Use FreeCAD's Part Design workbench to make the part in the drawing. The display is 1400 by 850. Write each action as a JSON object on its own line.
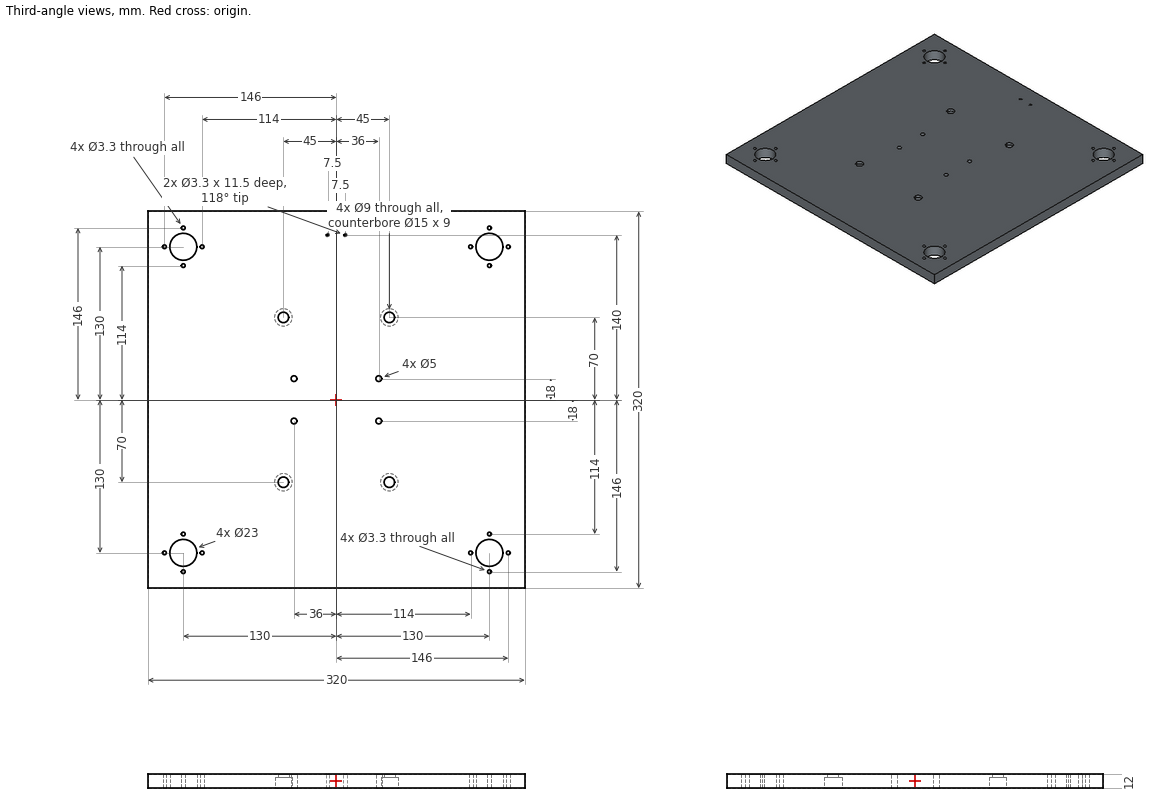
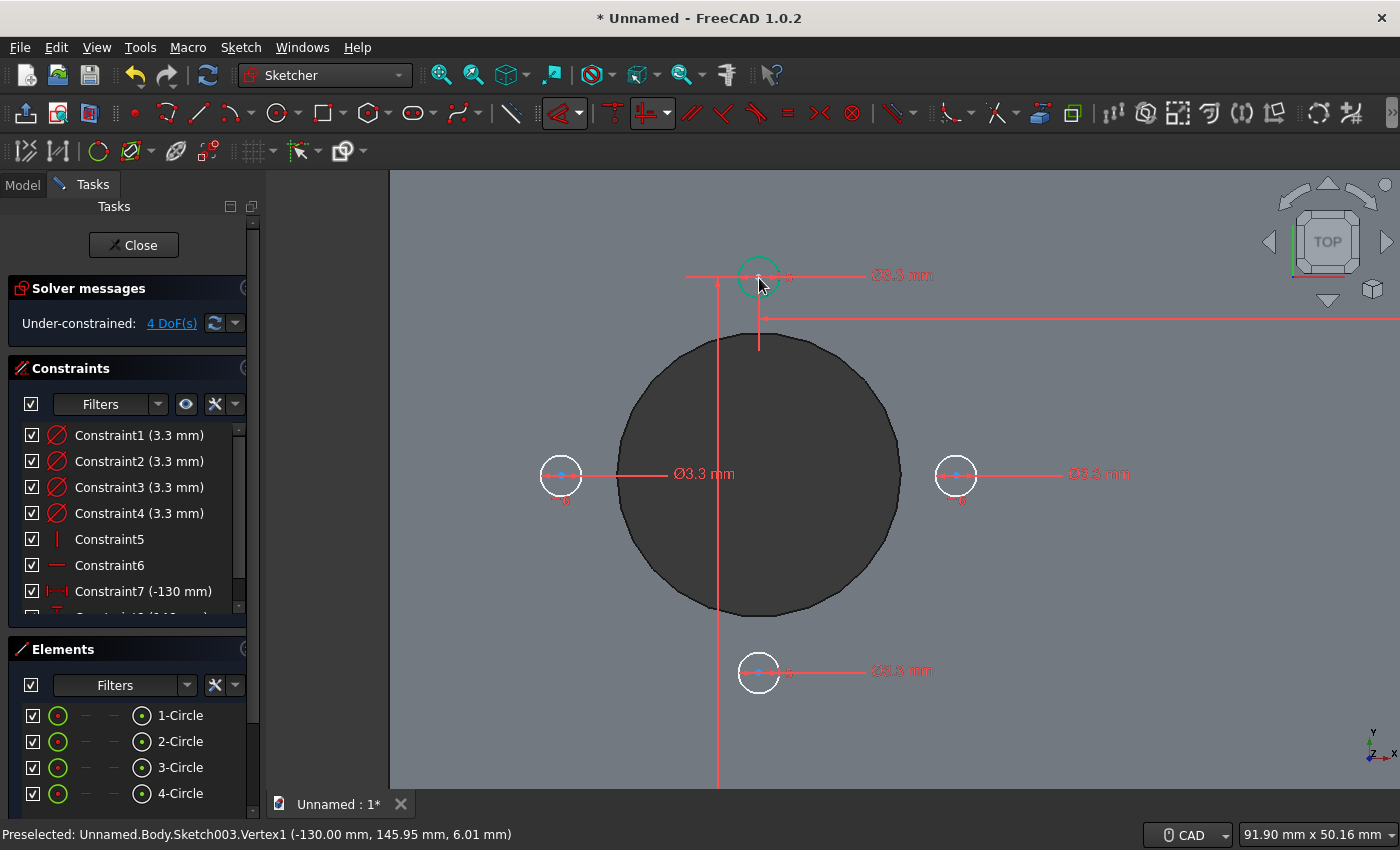
{"action": "left_click", "coordinate": [956, 476]}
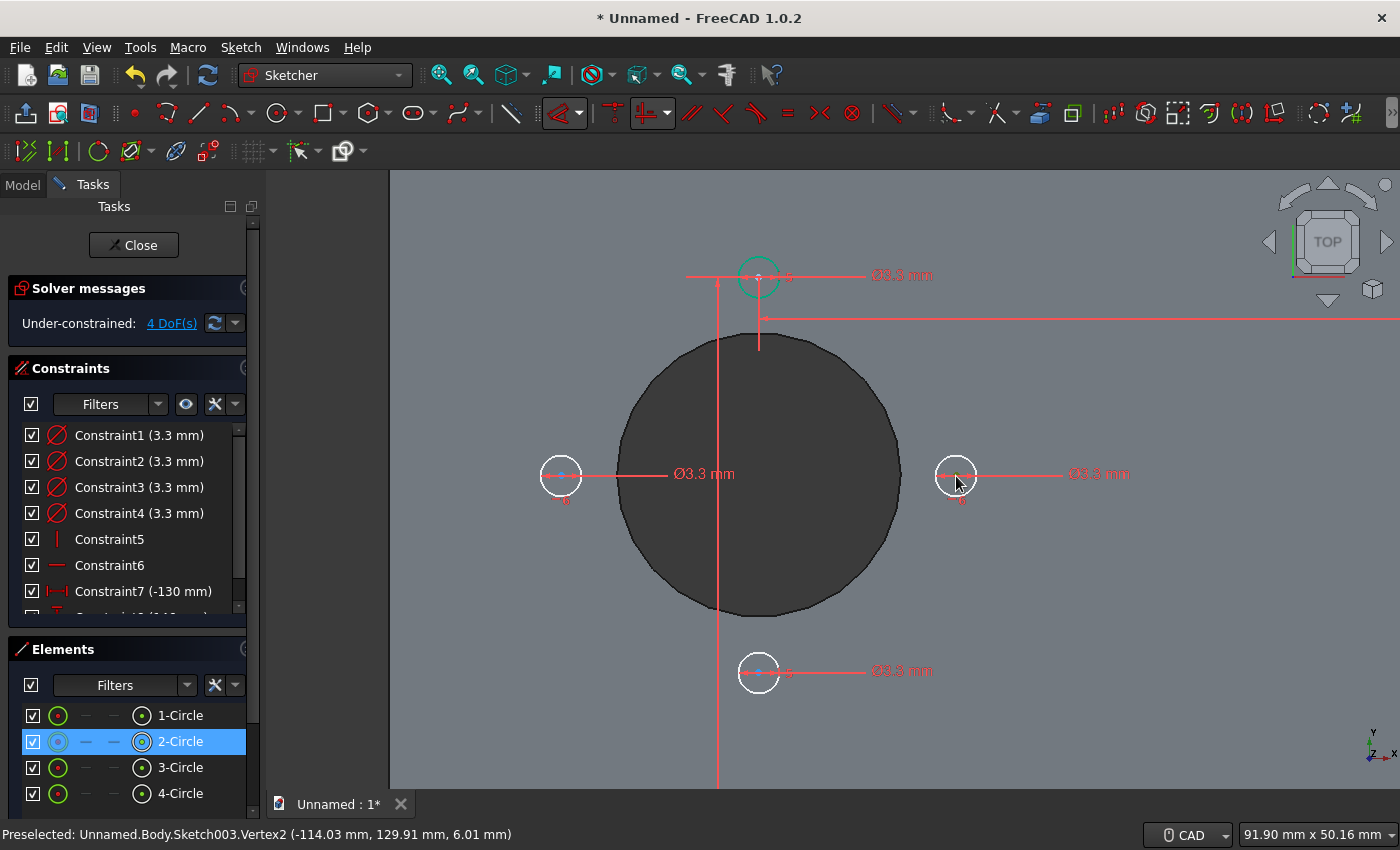
{"action": "left_click", "coordinate": [582, 114]}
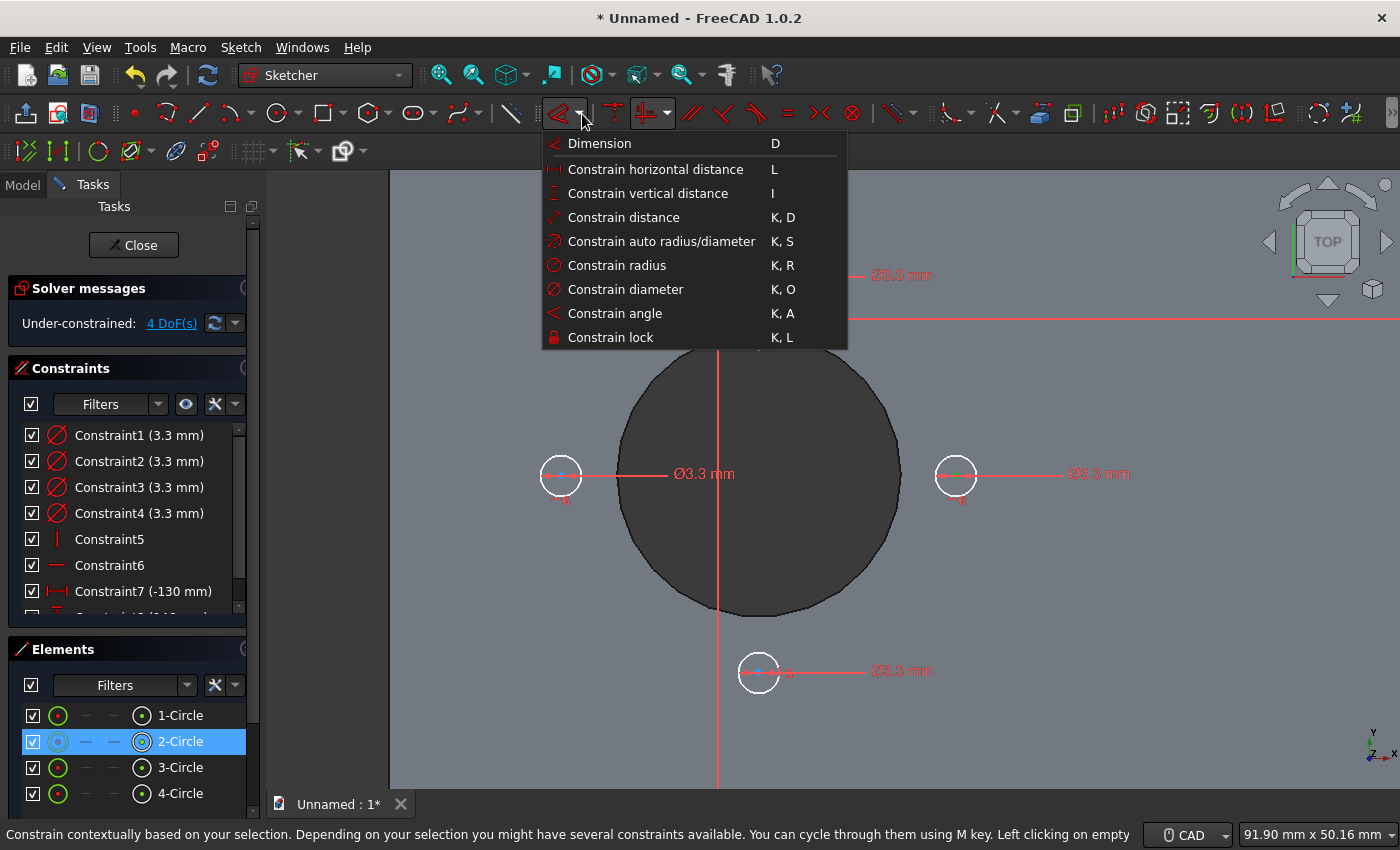
{"action": "left_click", "coordinate": [695, 169]}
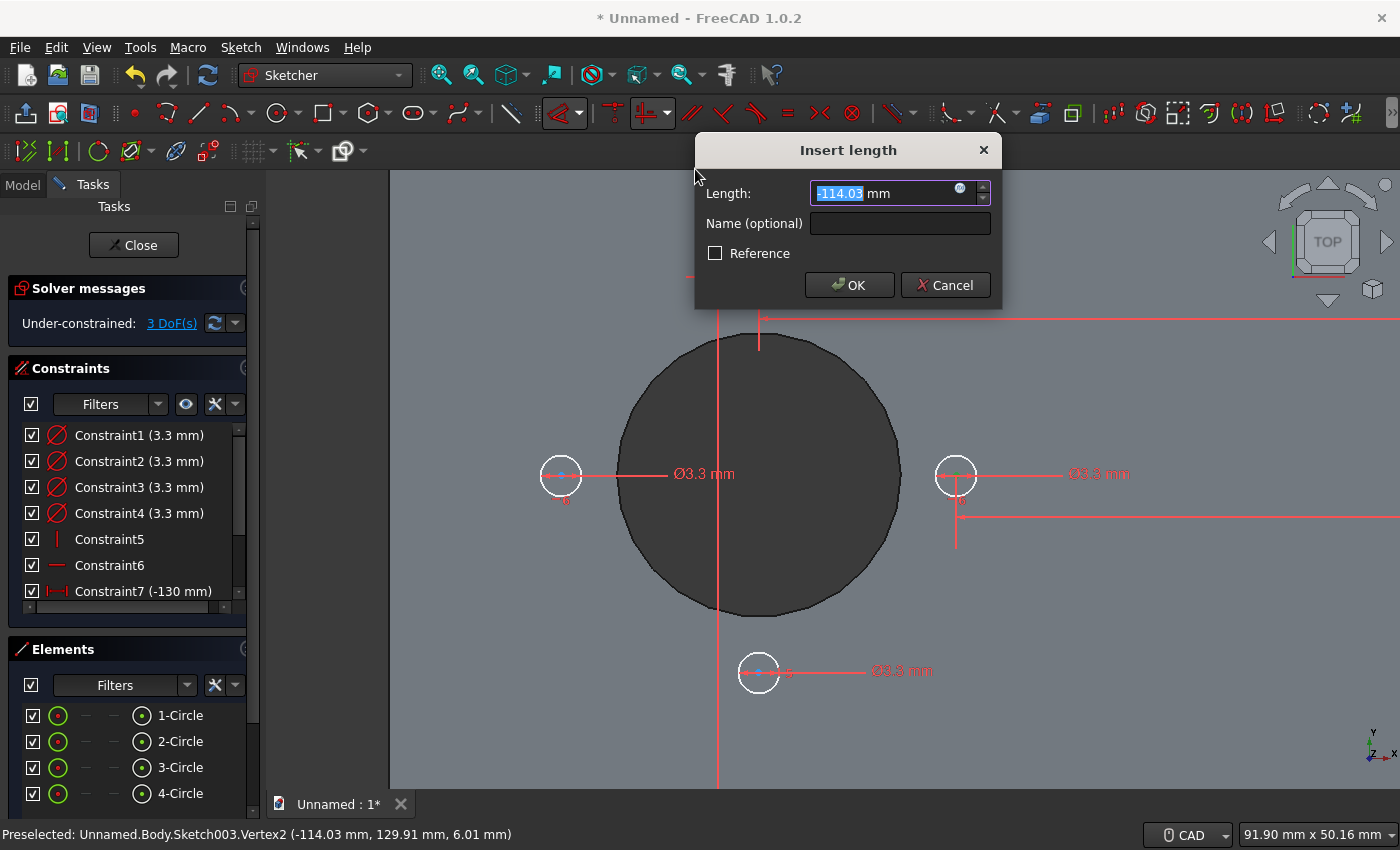
{"action": "type", "text": "-114"}
{"action": "key", "text": "Return"}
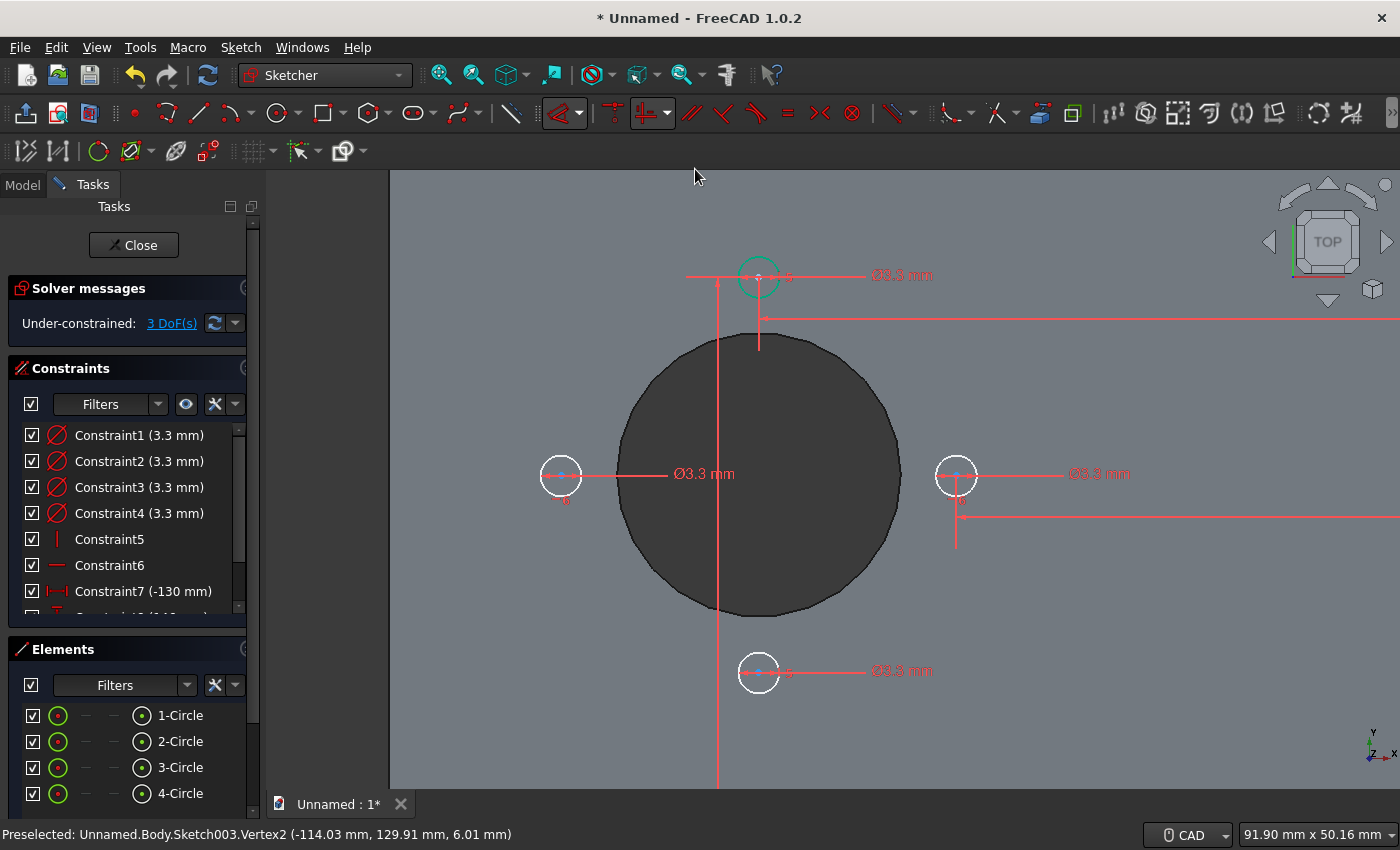
{"action": "left_click", "coordinate": [956, 476]}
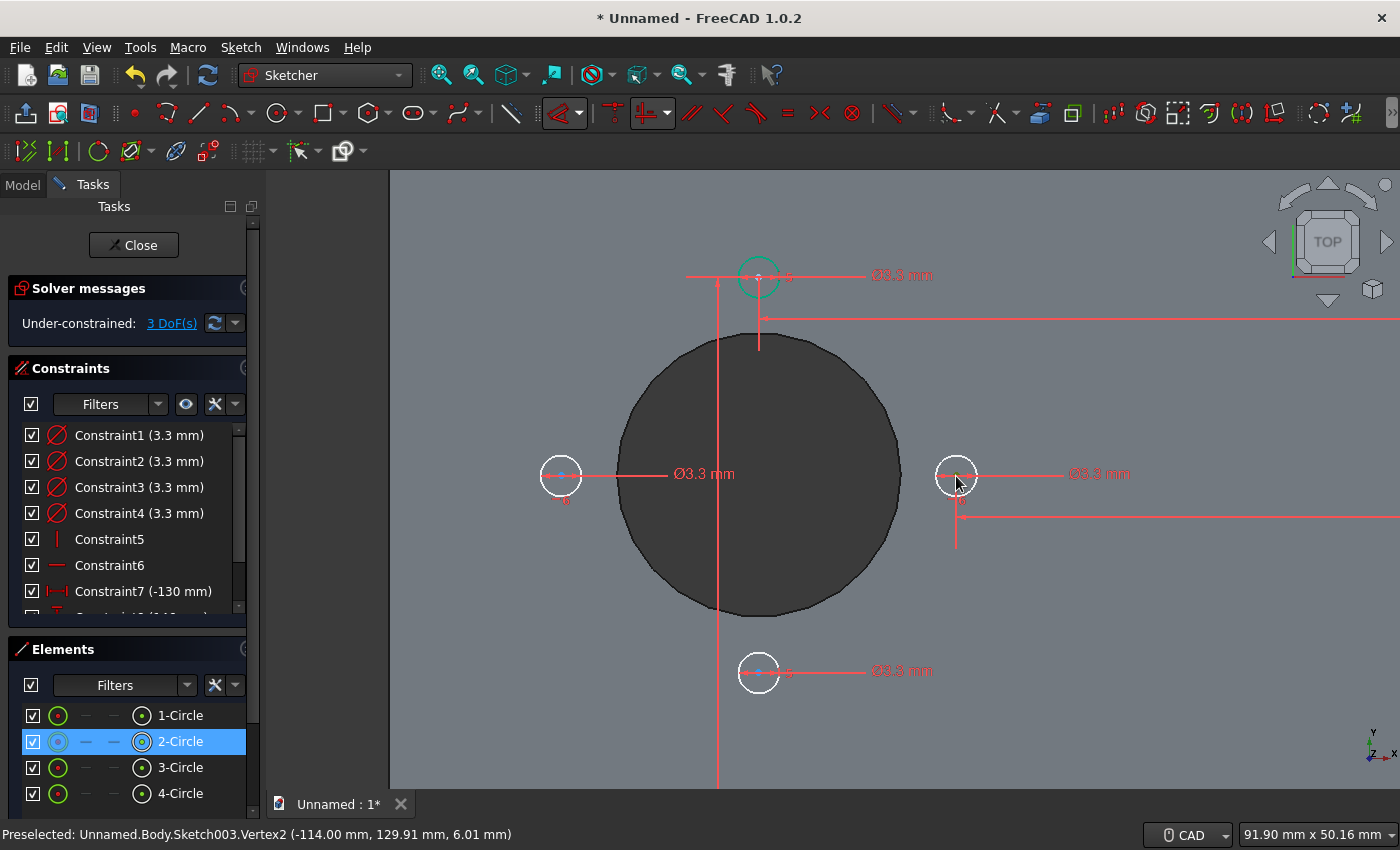
{"action": "left_click", "coordinate": [582, 114]}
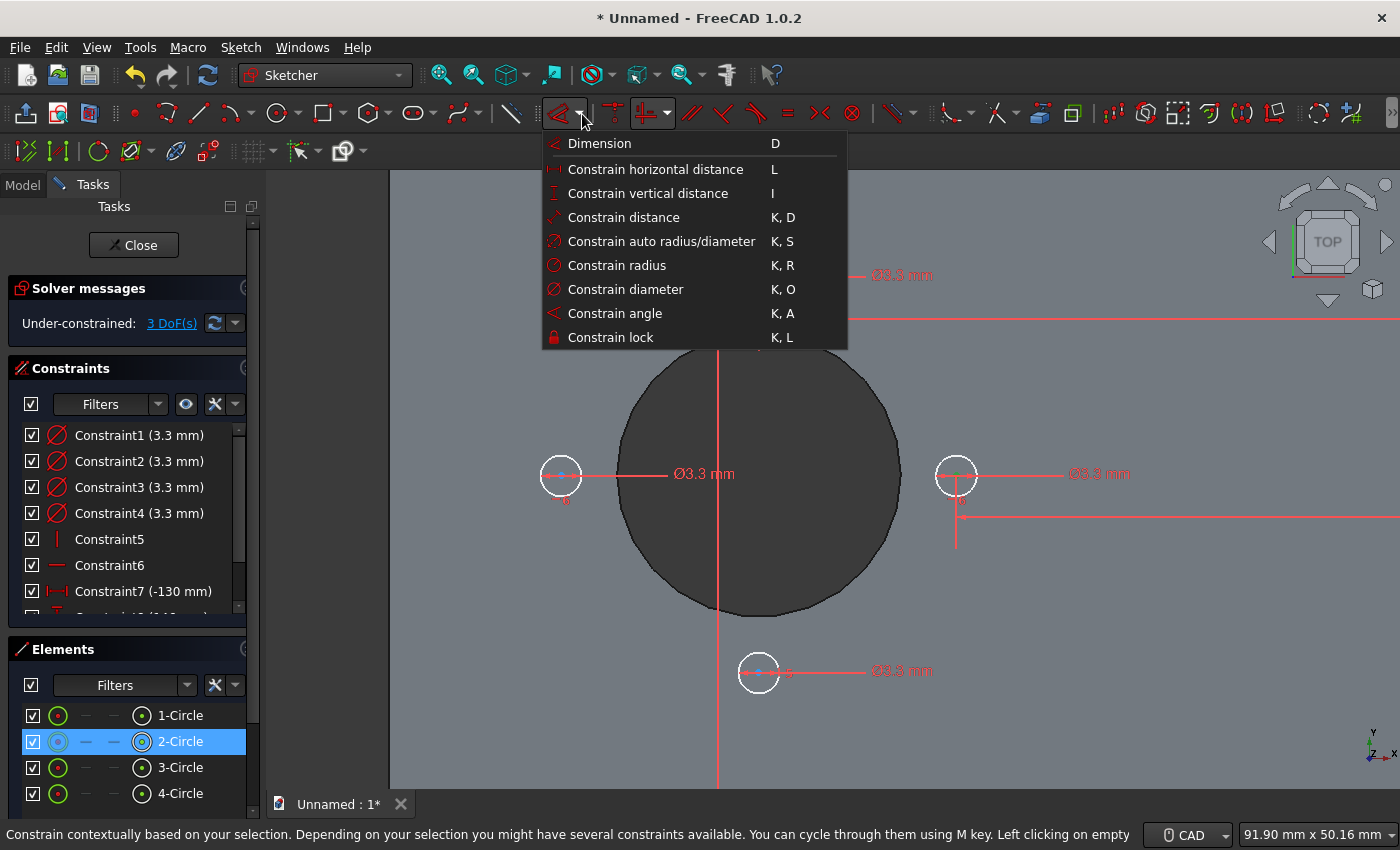
{"action": "left_click", "coordinate": [695, 193]}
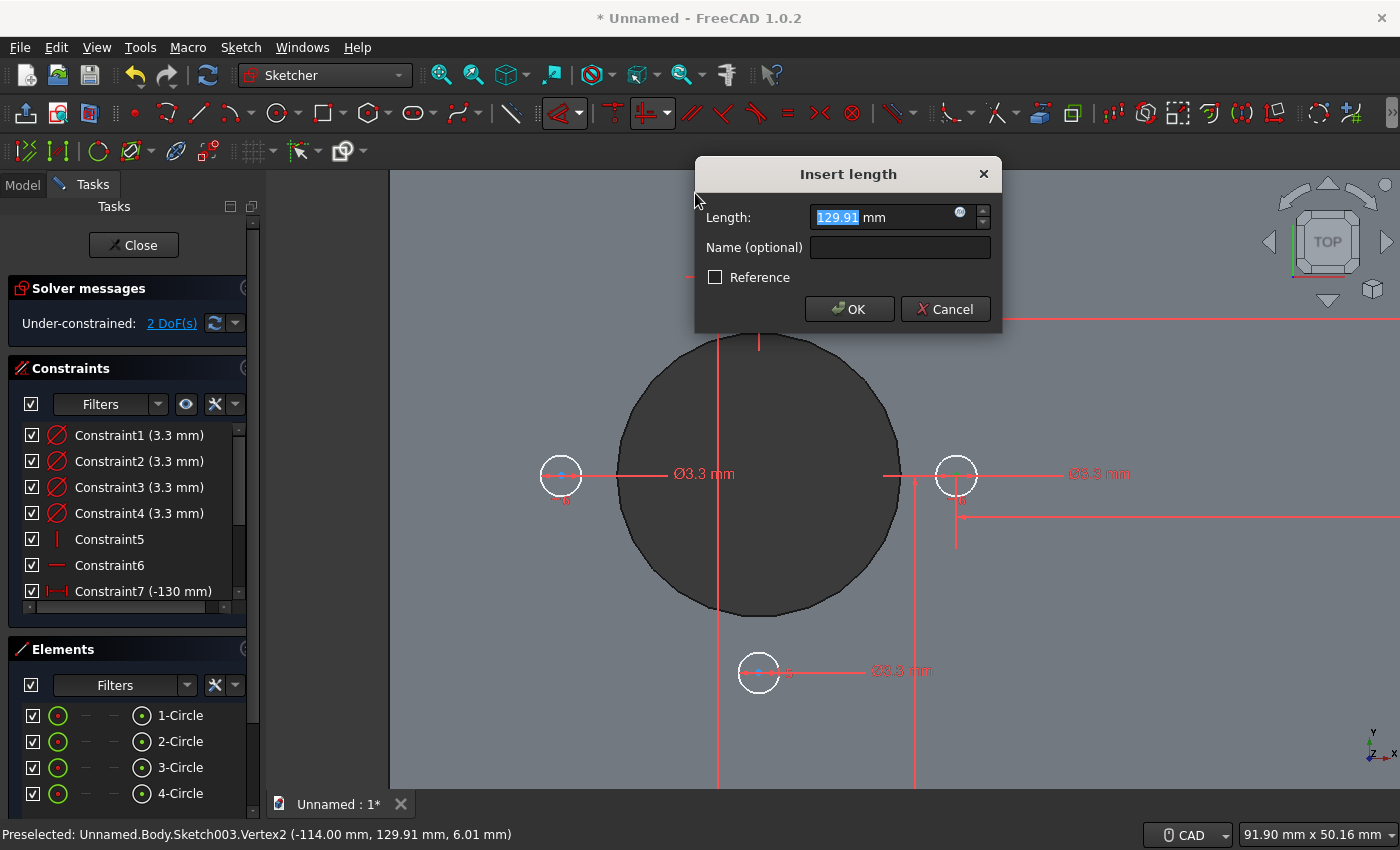
{"action": "type", "text": "130"}
{"action": "key", "text": "Return"}